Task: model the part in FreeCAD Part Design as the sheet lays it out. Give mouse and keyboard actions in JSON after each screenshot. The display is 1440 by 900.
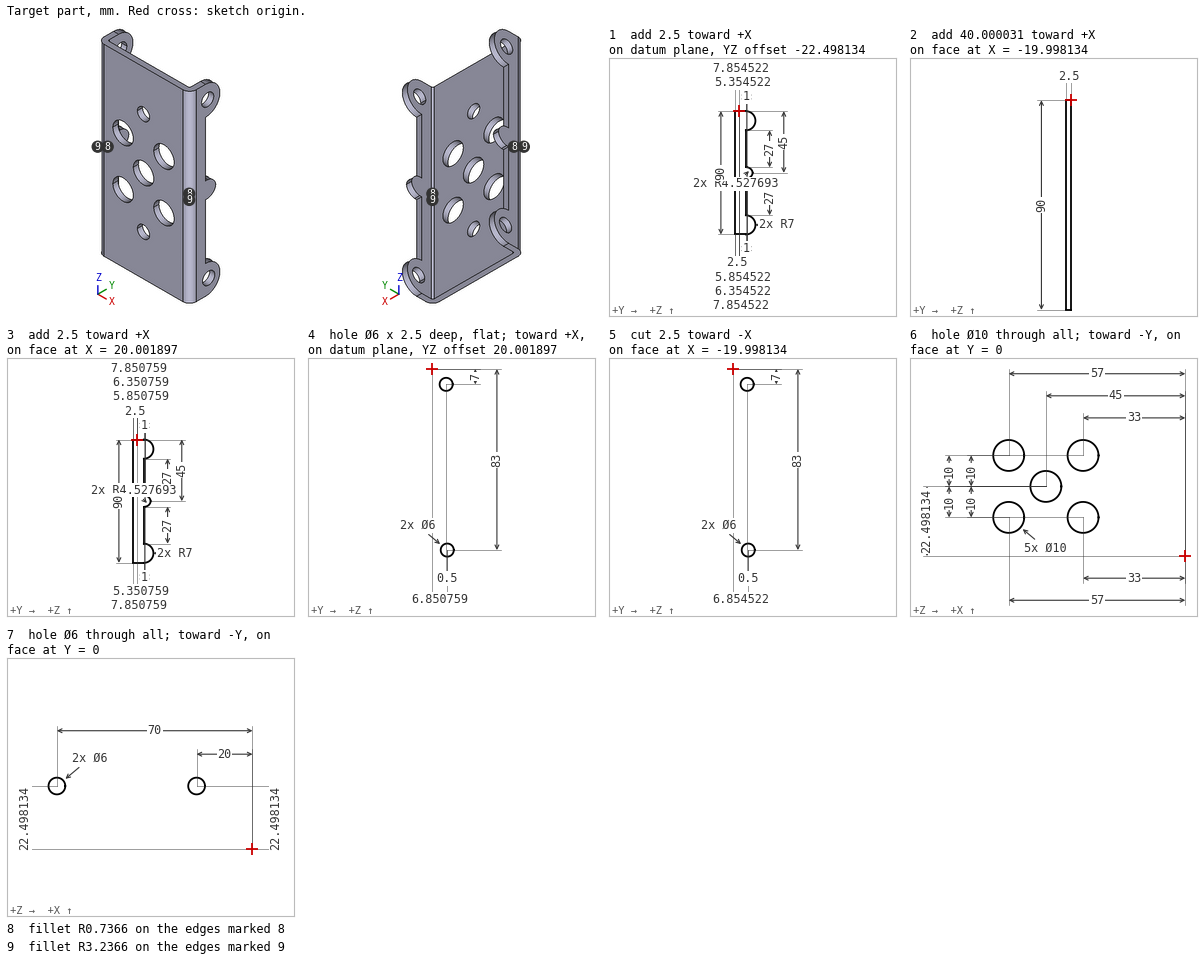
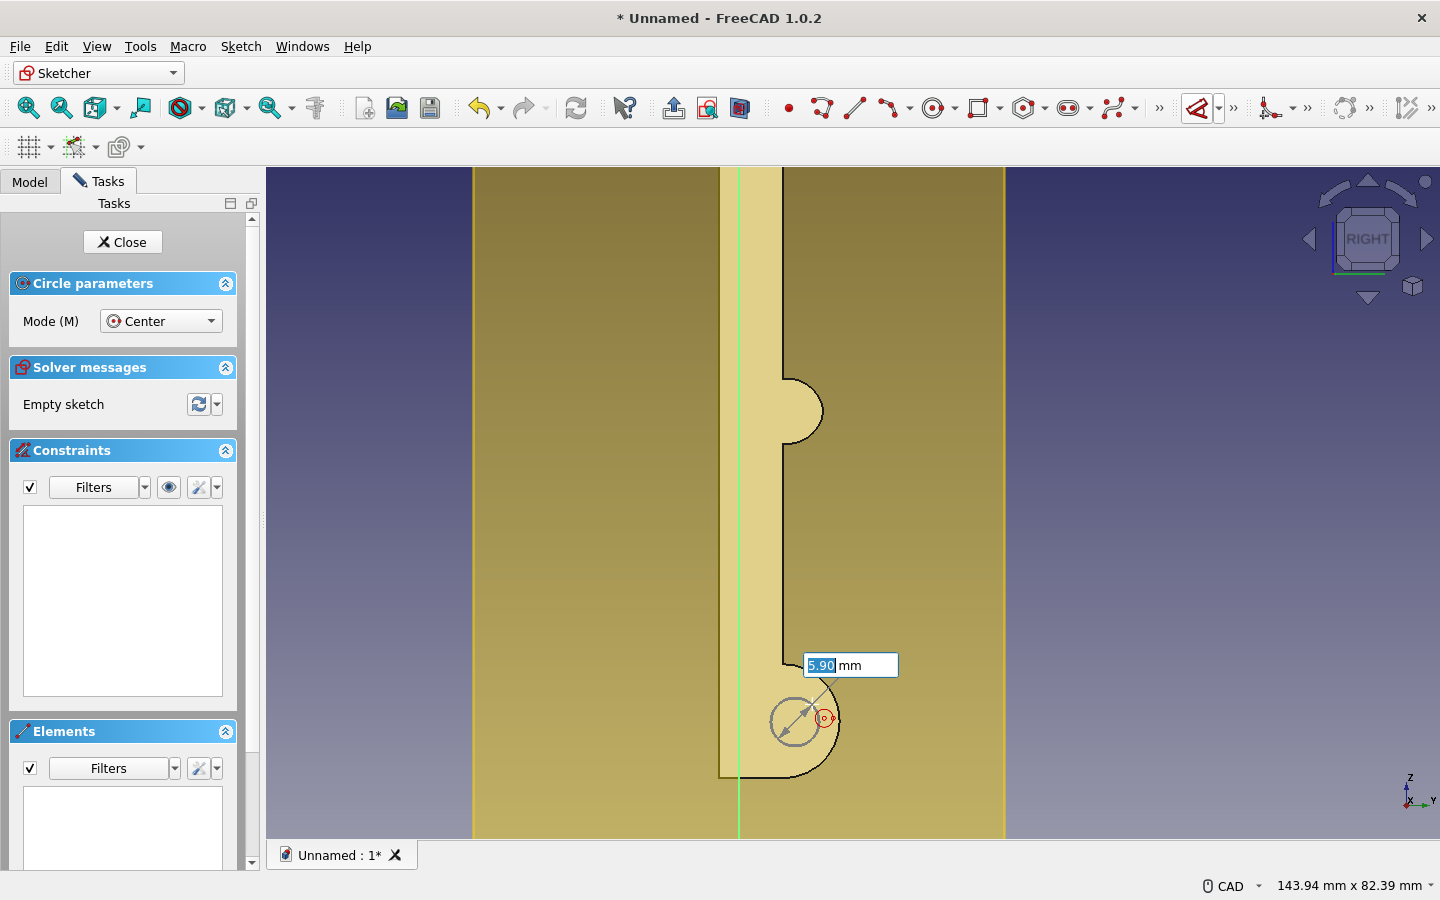
{"action": "type", "text": "6"}
{"action": "key", "text": "Return"}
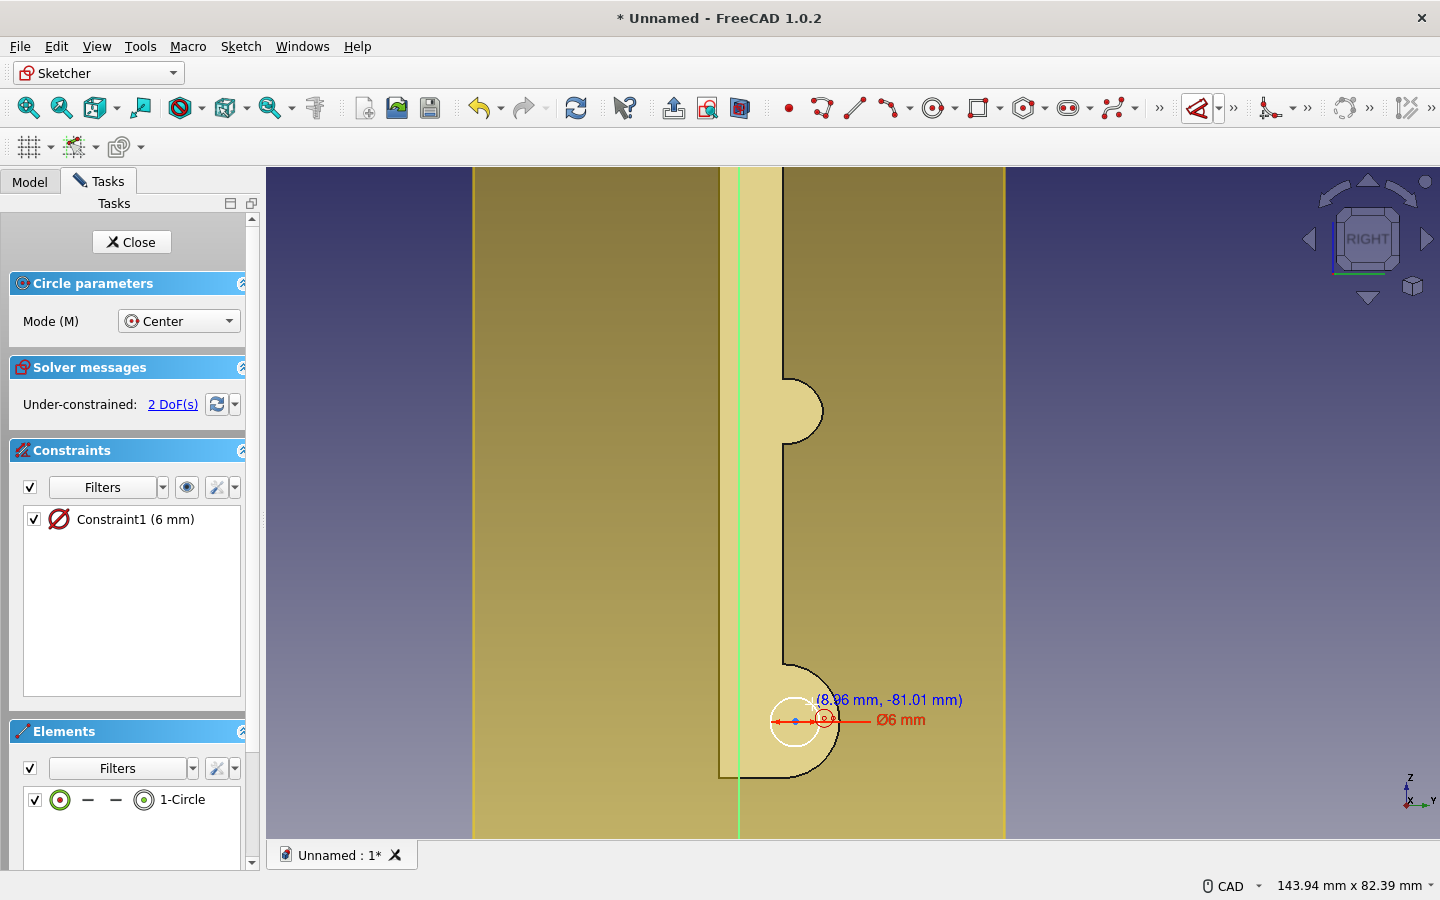
{"action": "scroll", "coordinate": [795, 723], "scroll_direction": "down", "scroll_amount": 2}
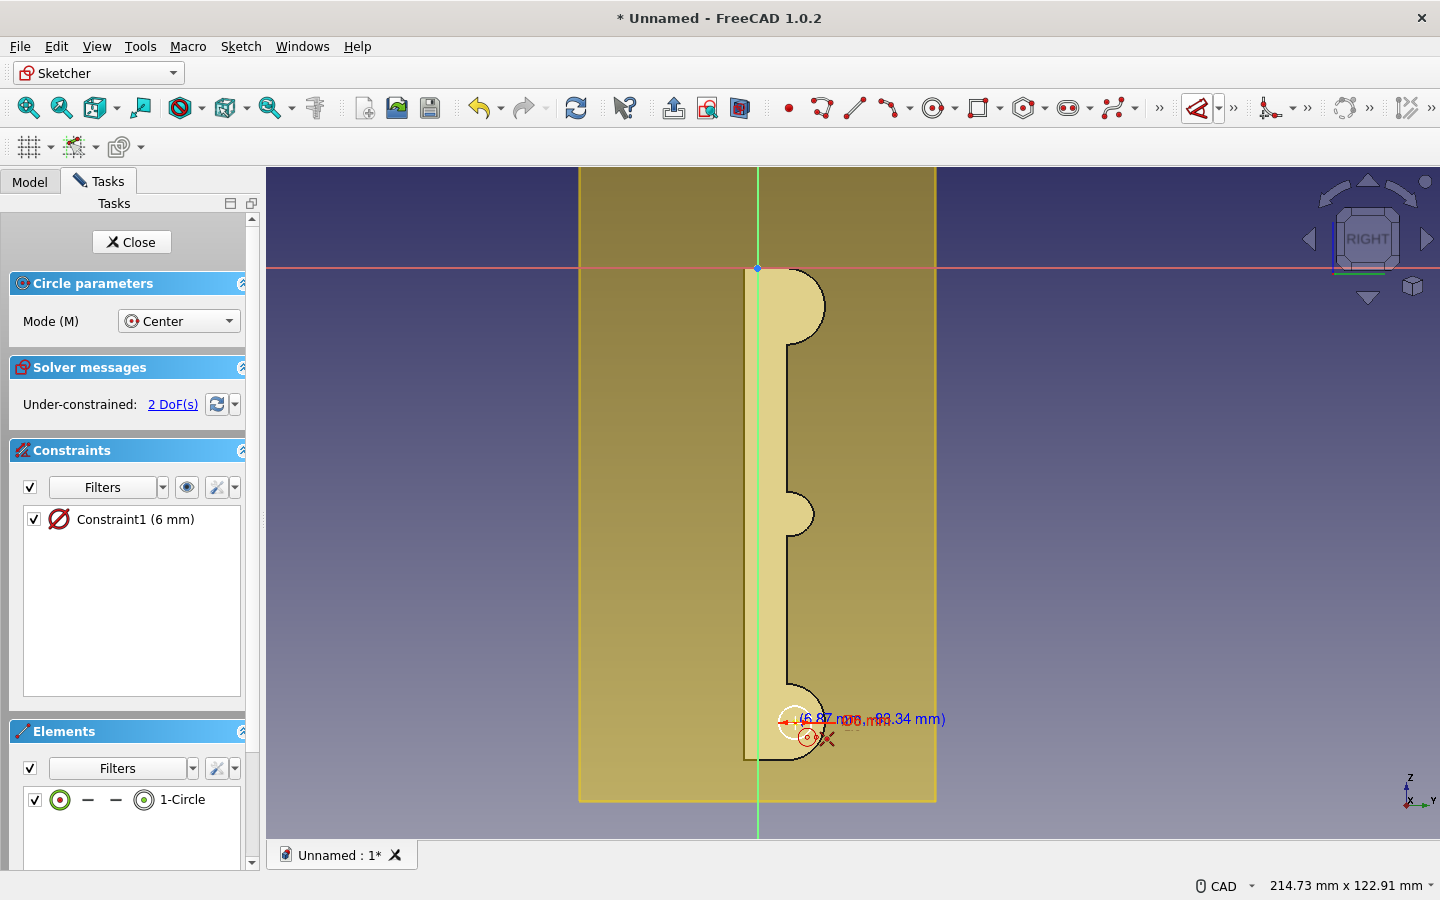
{"action": "scroll", "coordinate": [792, 307], "scroll_direction": "up", "scroll_amount": 2}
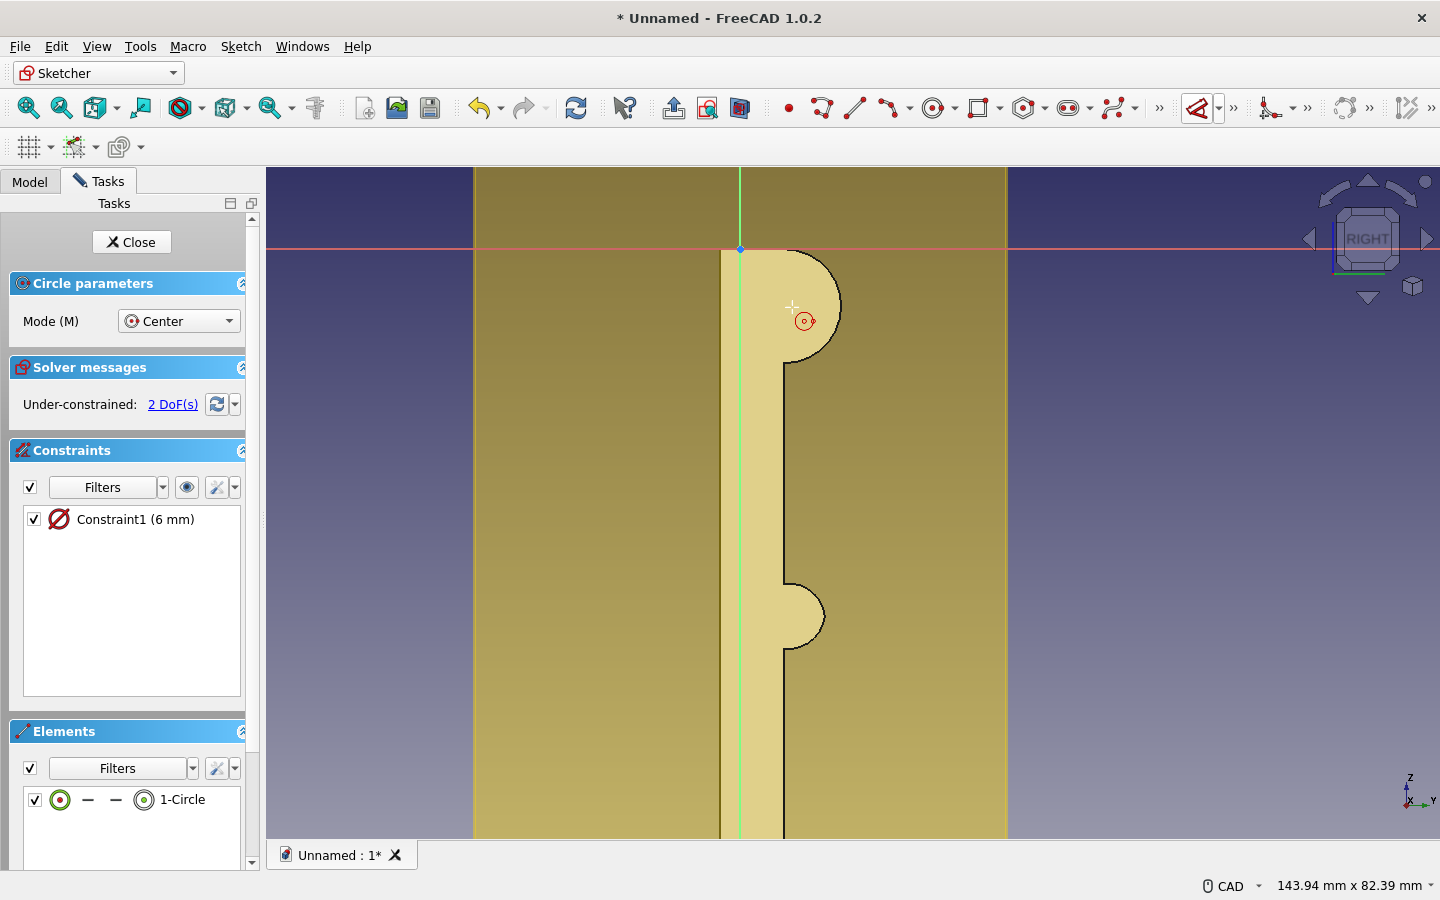
{"action": "left_click", "coordinate": [792, 306]}
{"action": "mouse_move", "coordinate": [810, 289]}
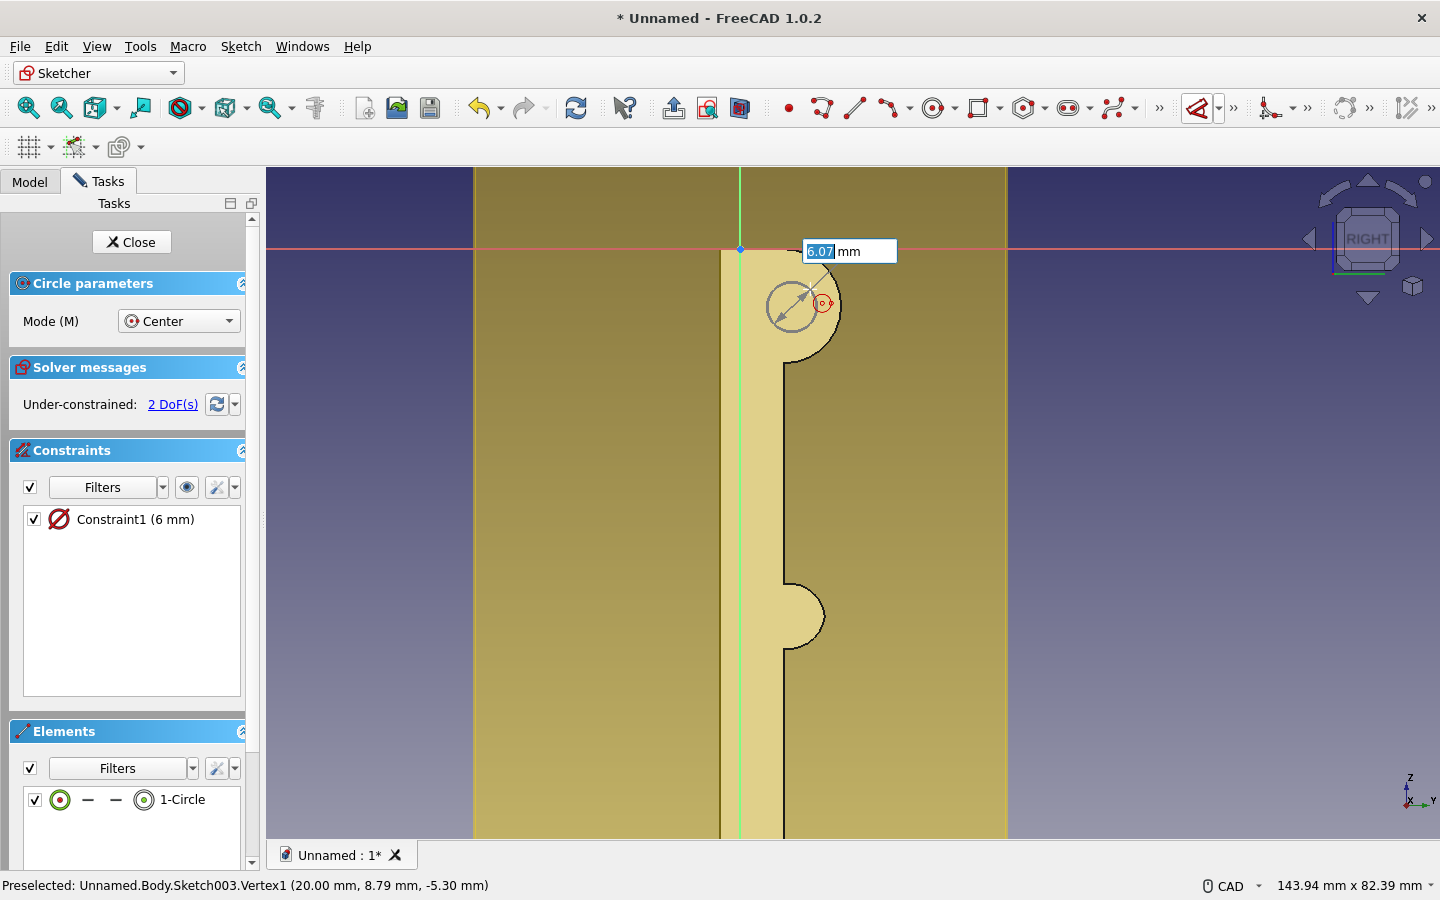
{"action": "type", "text": "6"}
{"action": "key", "text": "Return"}
{"action": "key", "text": "Escape"}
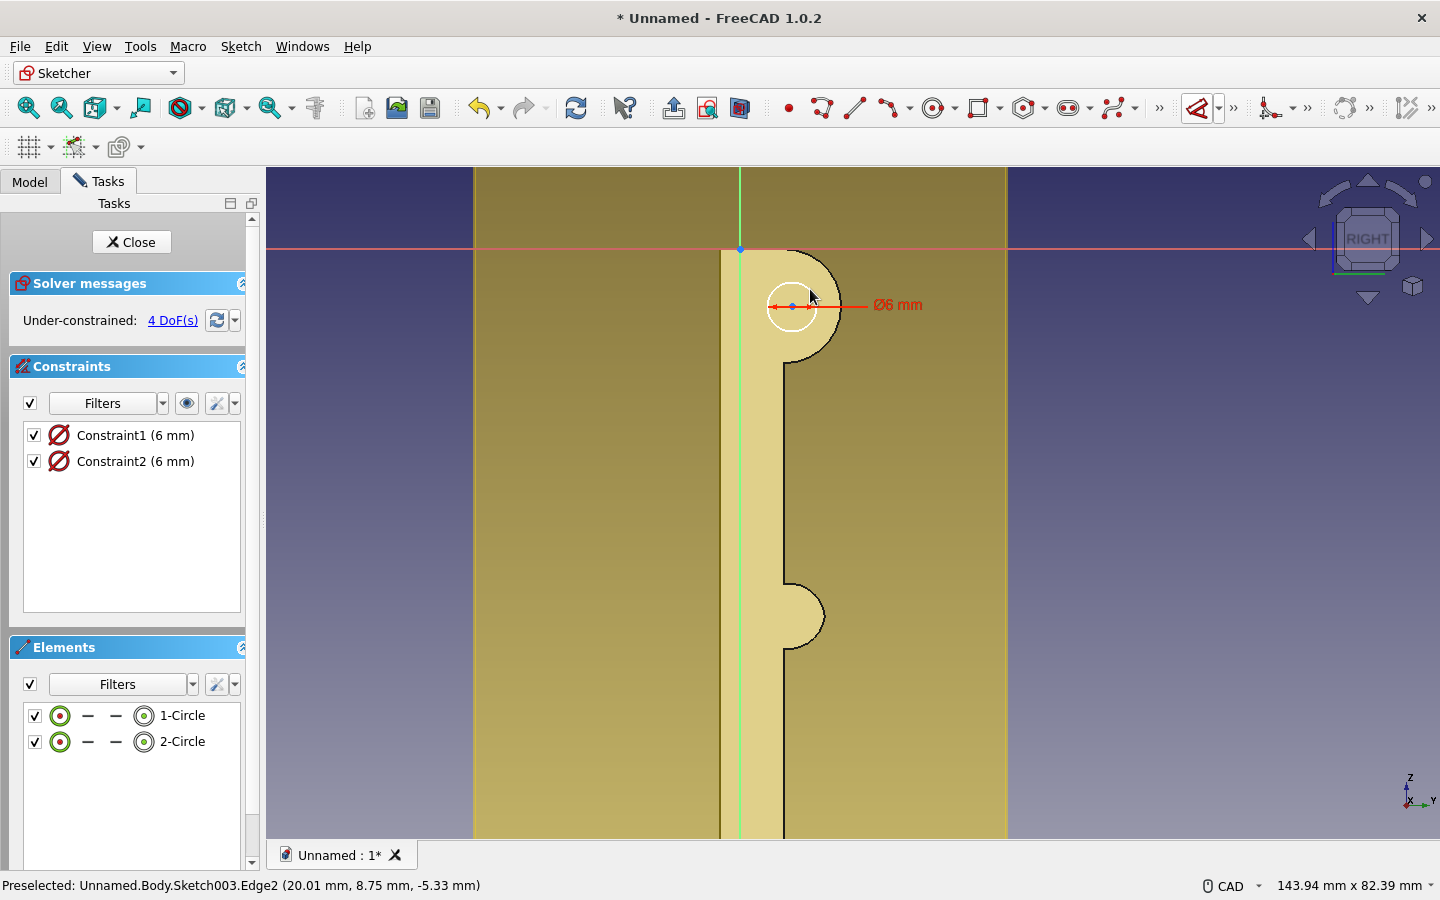
{"action": "left_click", "coordinate": [792, 307]}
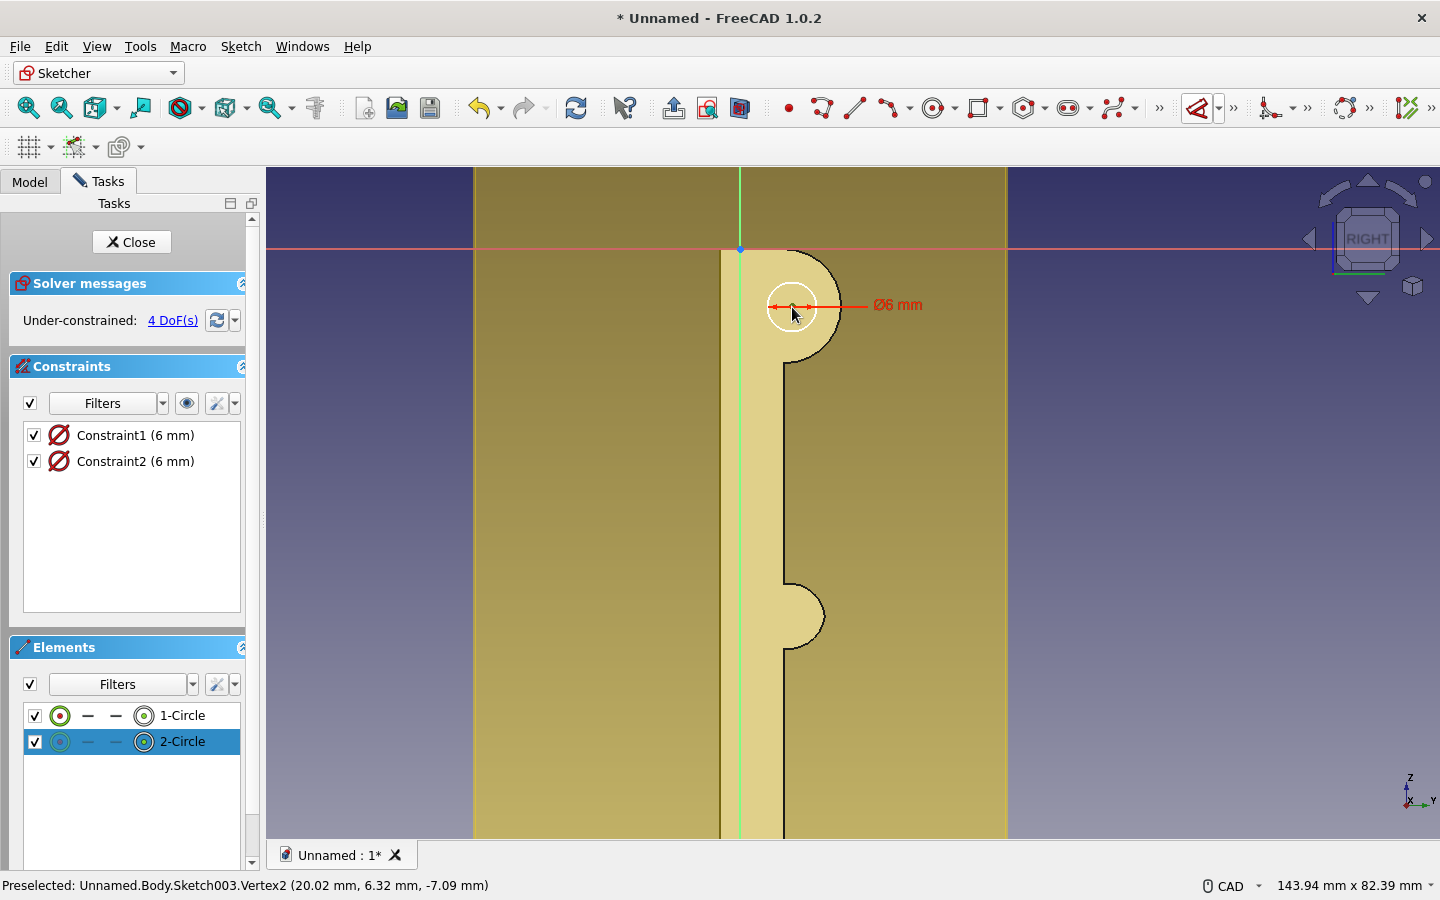
{"action": "key", "text": "i"}